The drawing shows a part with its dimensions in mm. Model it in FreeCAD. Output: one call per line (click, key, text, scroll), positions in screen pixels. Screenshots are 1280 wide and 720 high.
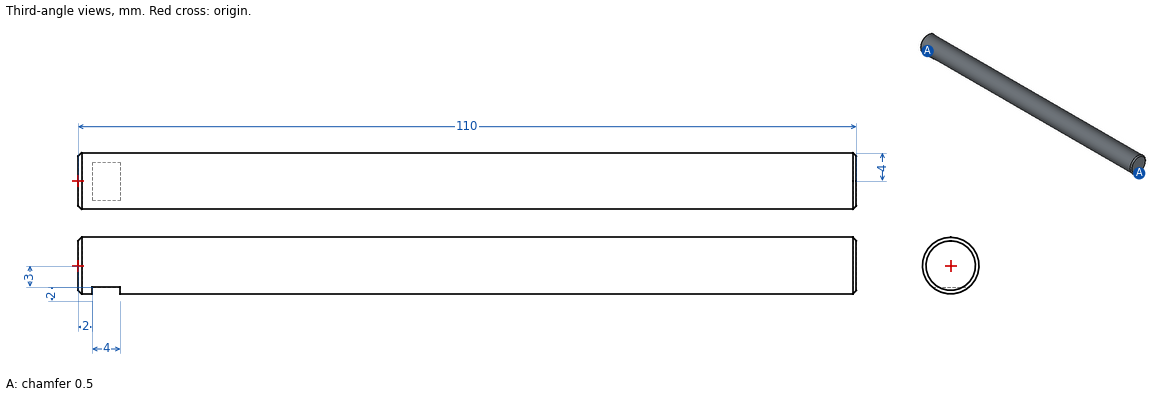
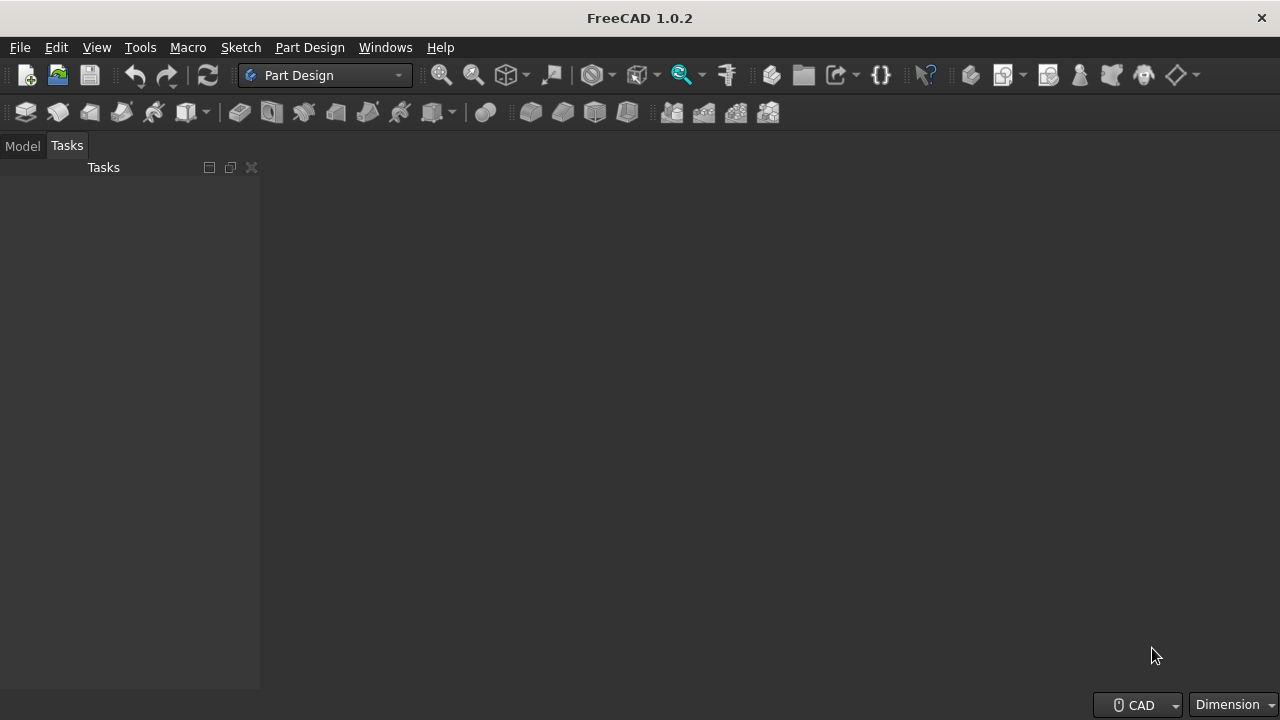
click(26, 76)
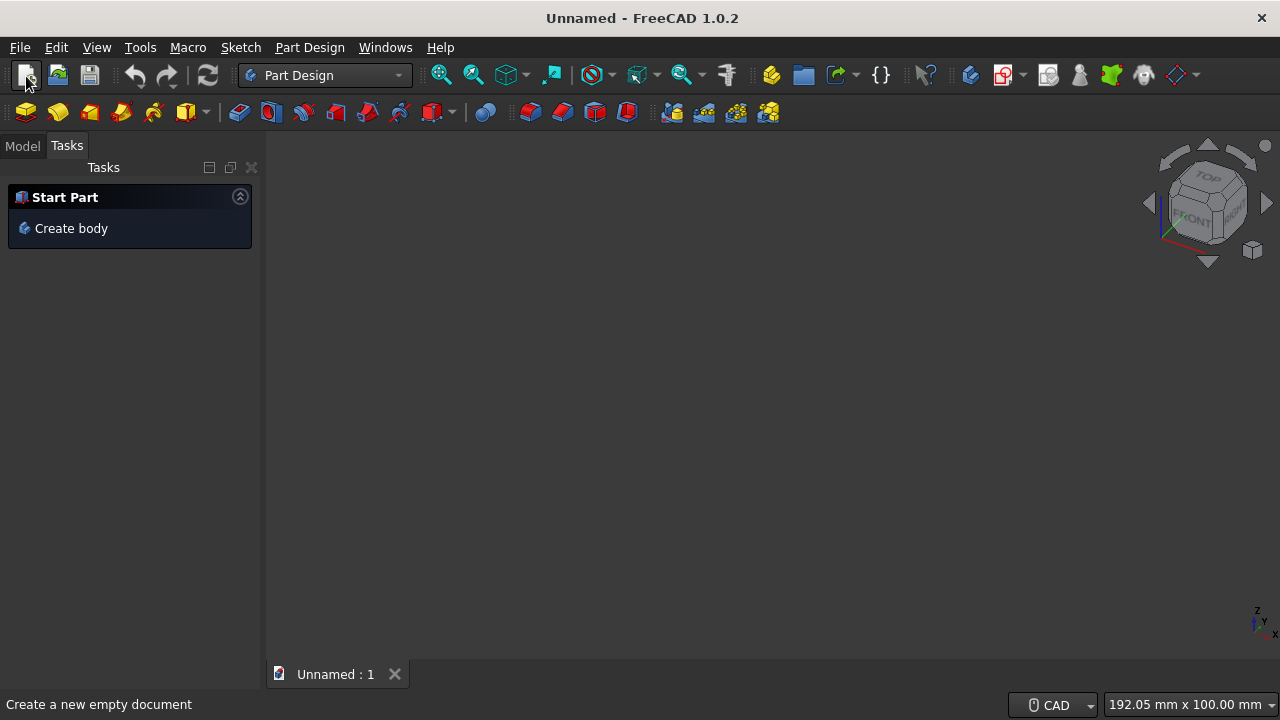
click(1004, 76)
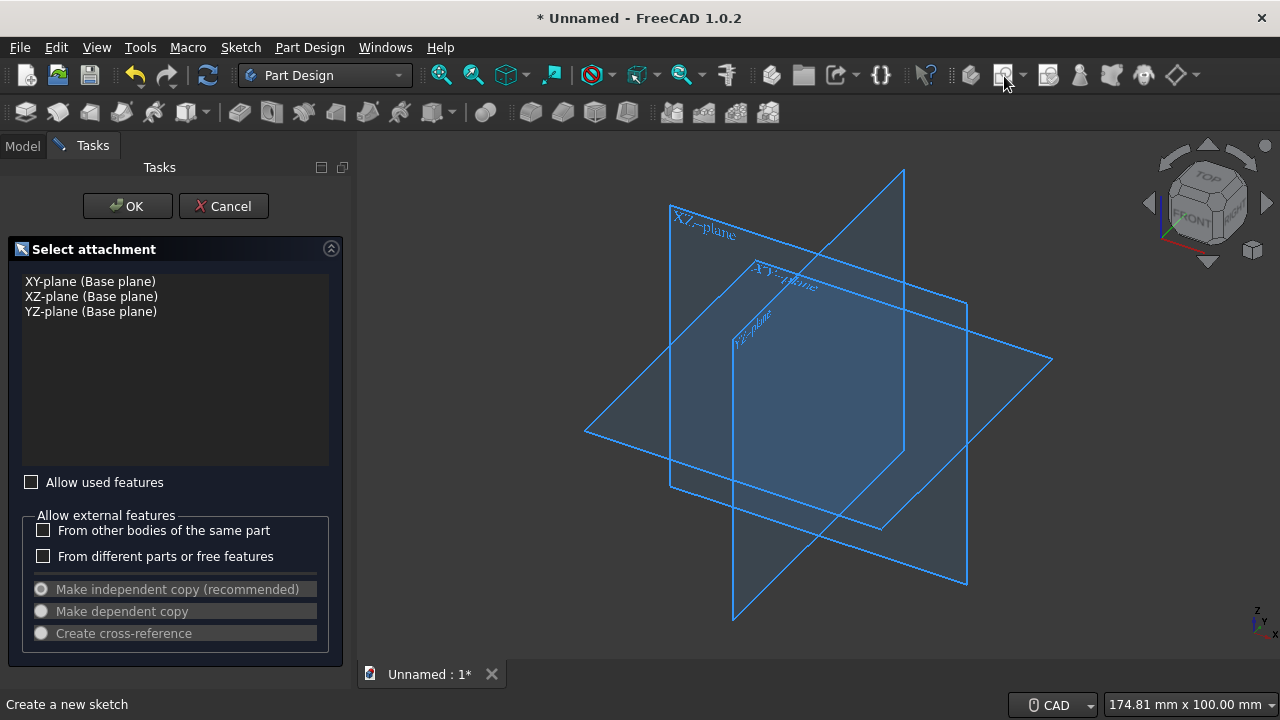
click(82, 282)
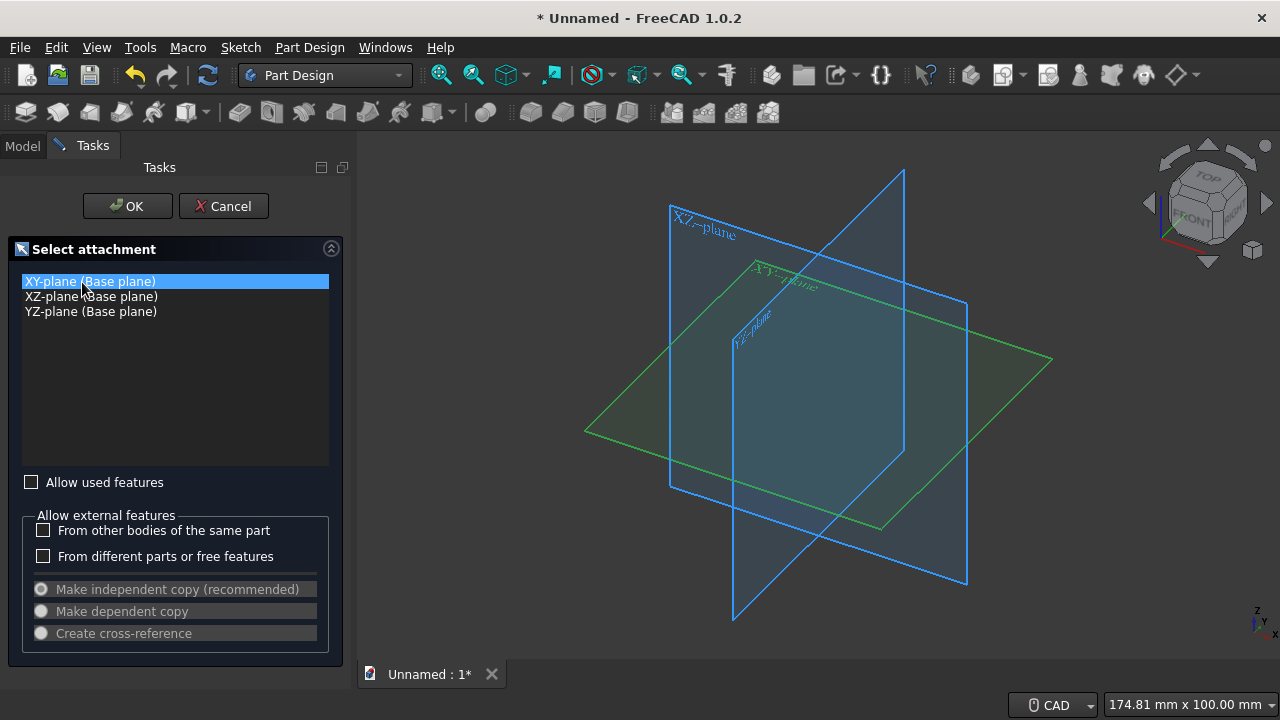
click(128, 206)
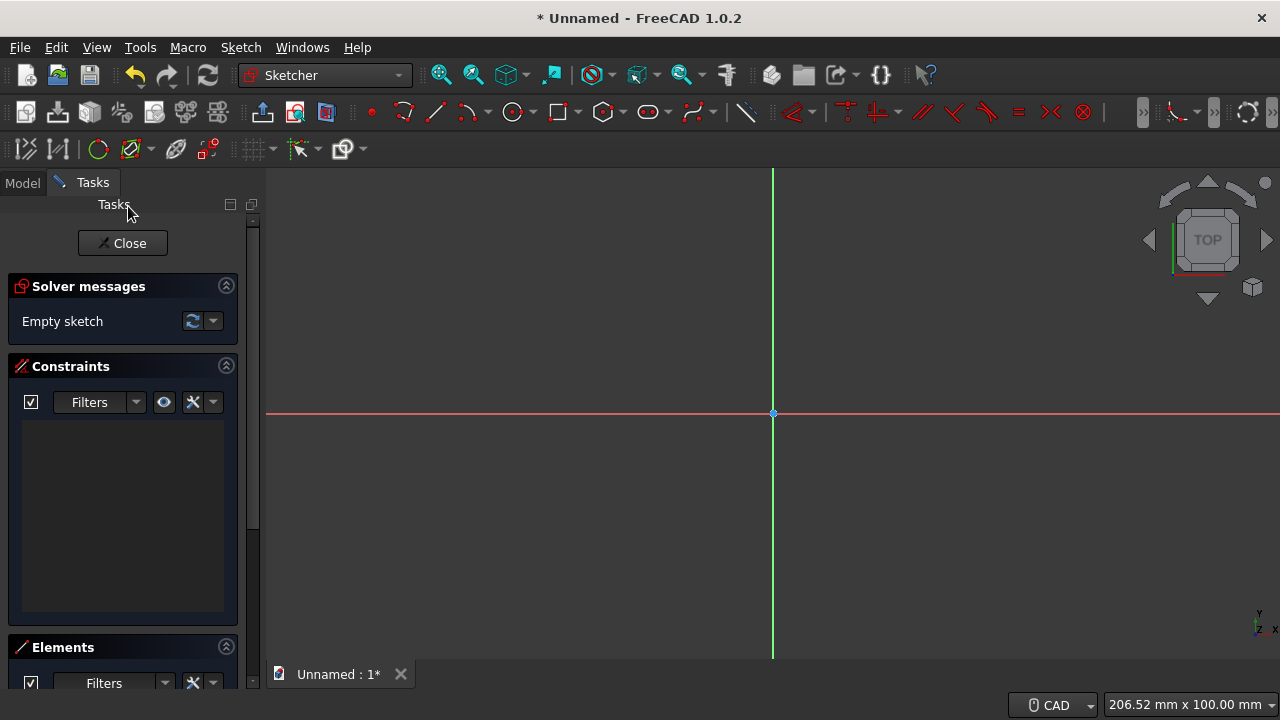
scroll(294, 433, down, 2)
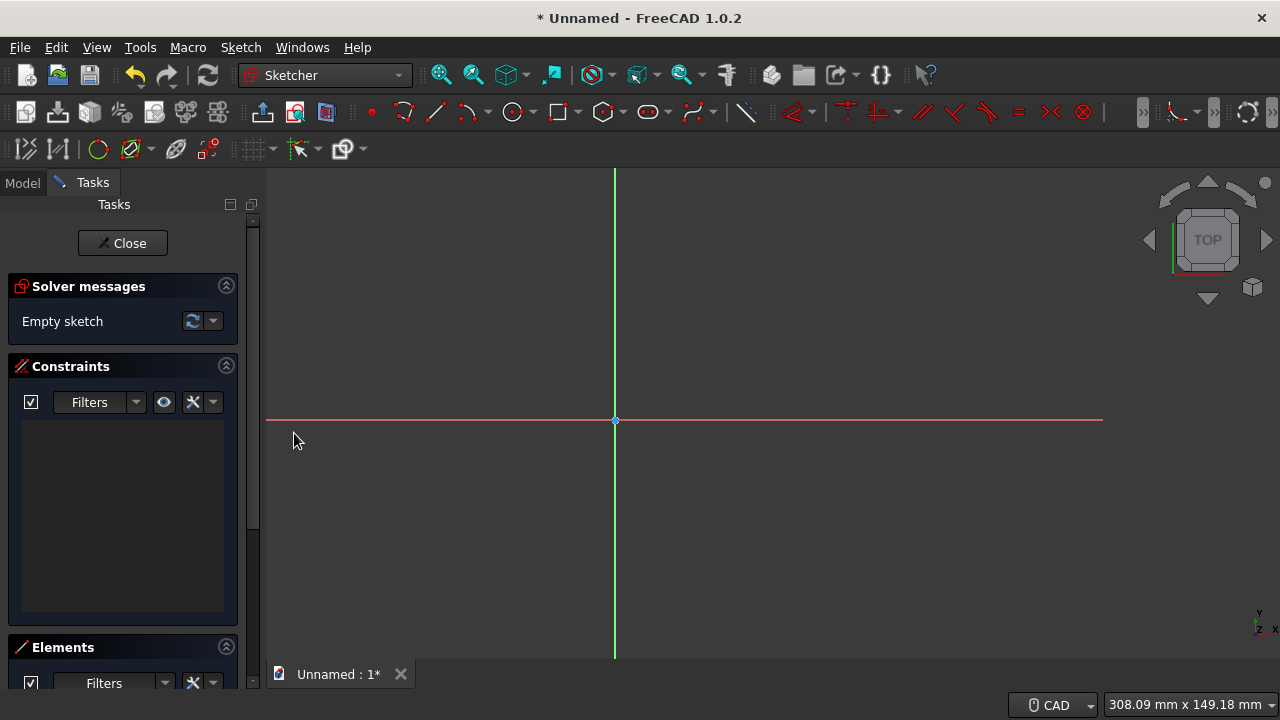
scroll(982, 414, up, 2)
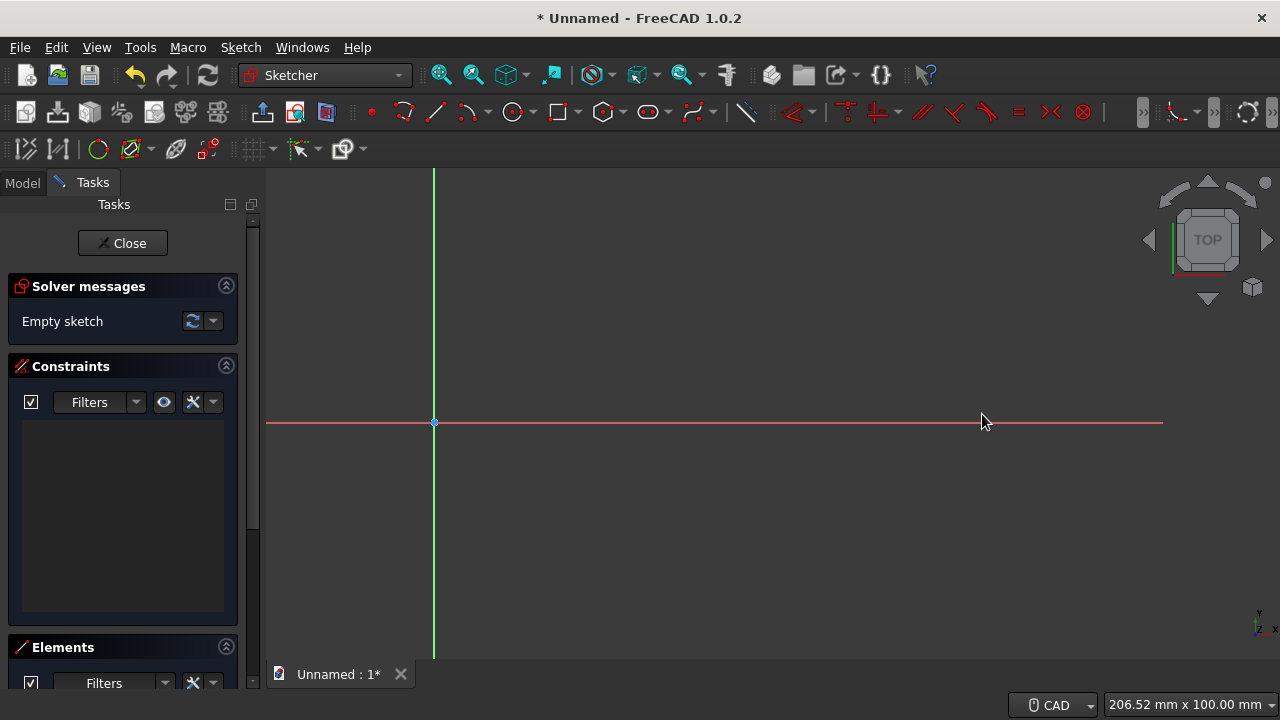
click(558, 112)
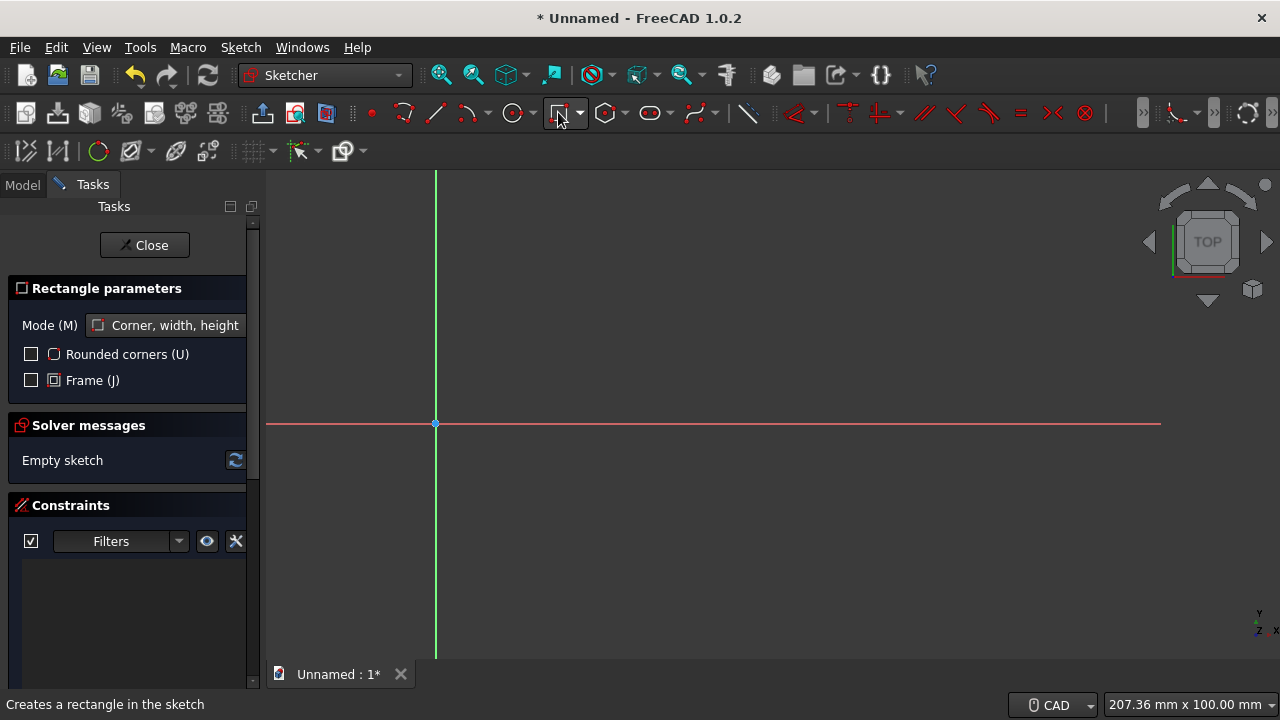
click(436, 424)
click(974, 404)
key(Escape)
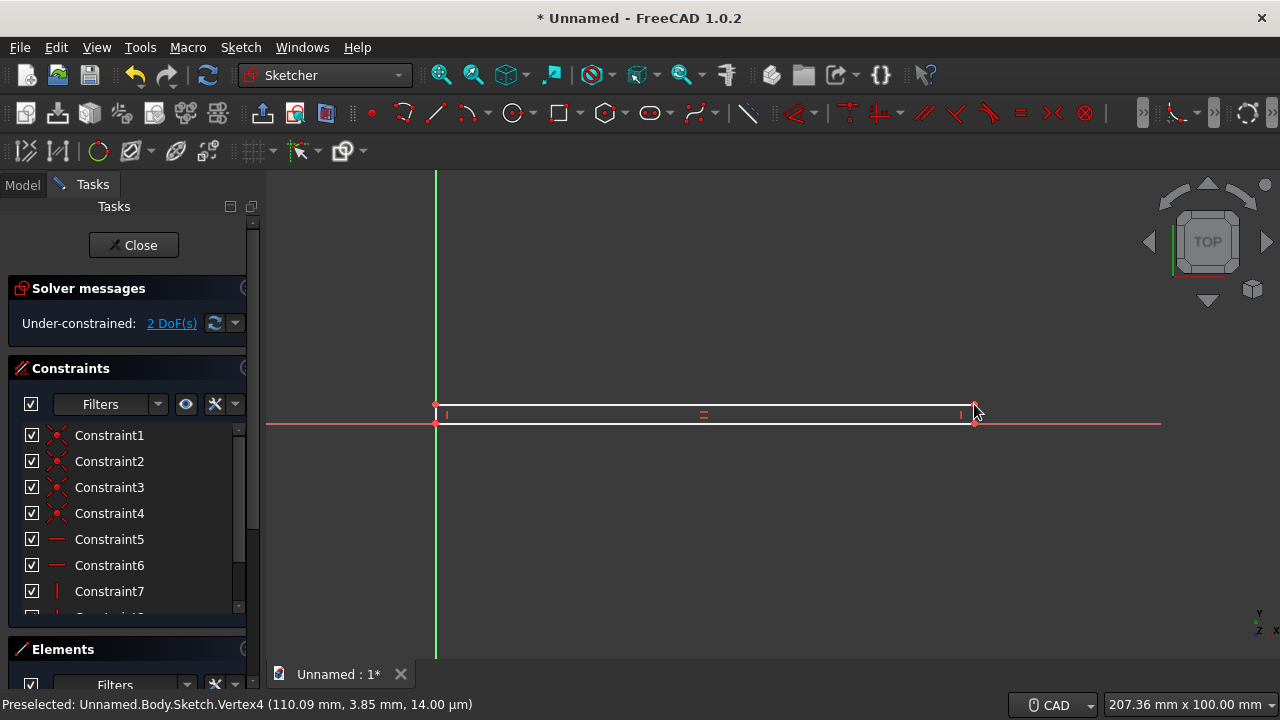
key(d)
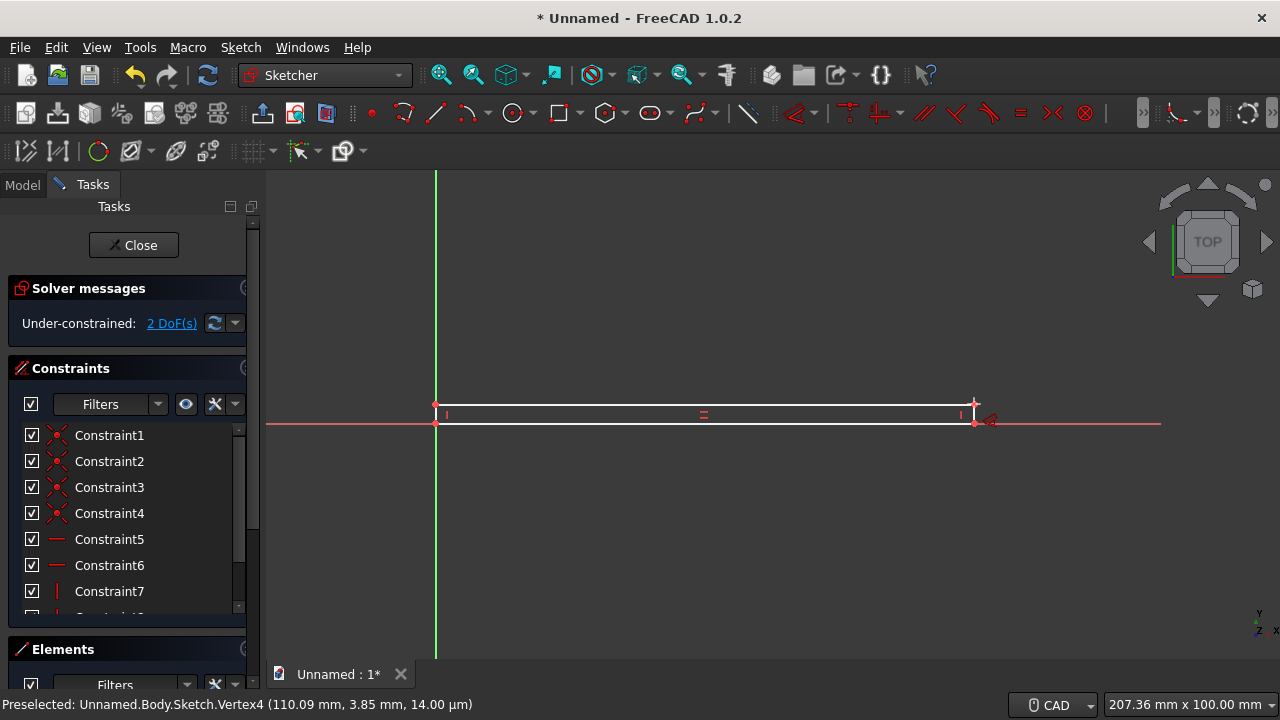
scroll(974, 414, up, 4)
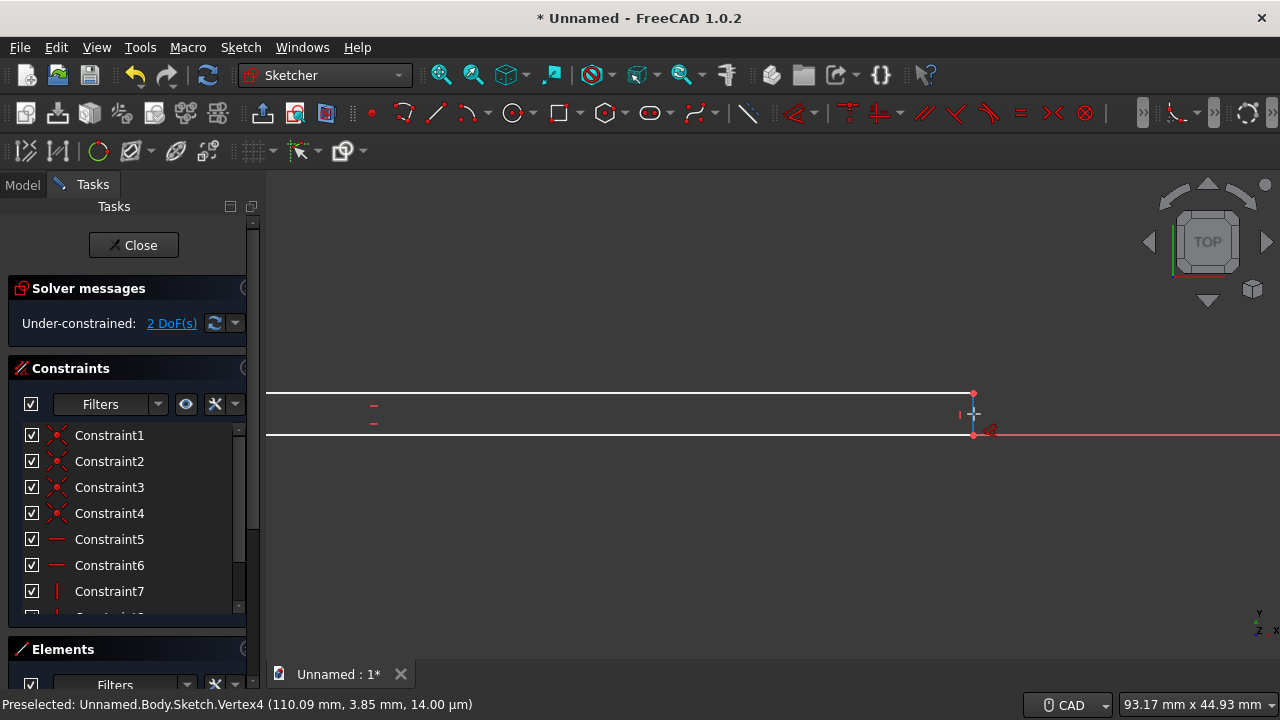
click(973, 414)
click(1007, 414)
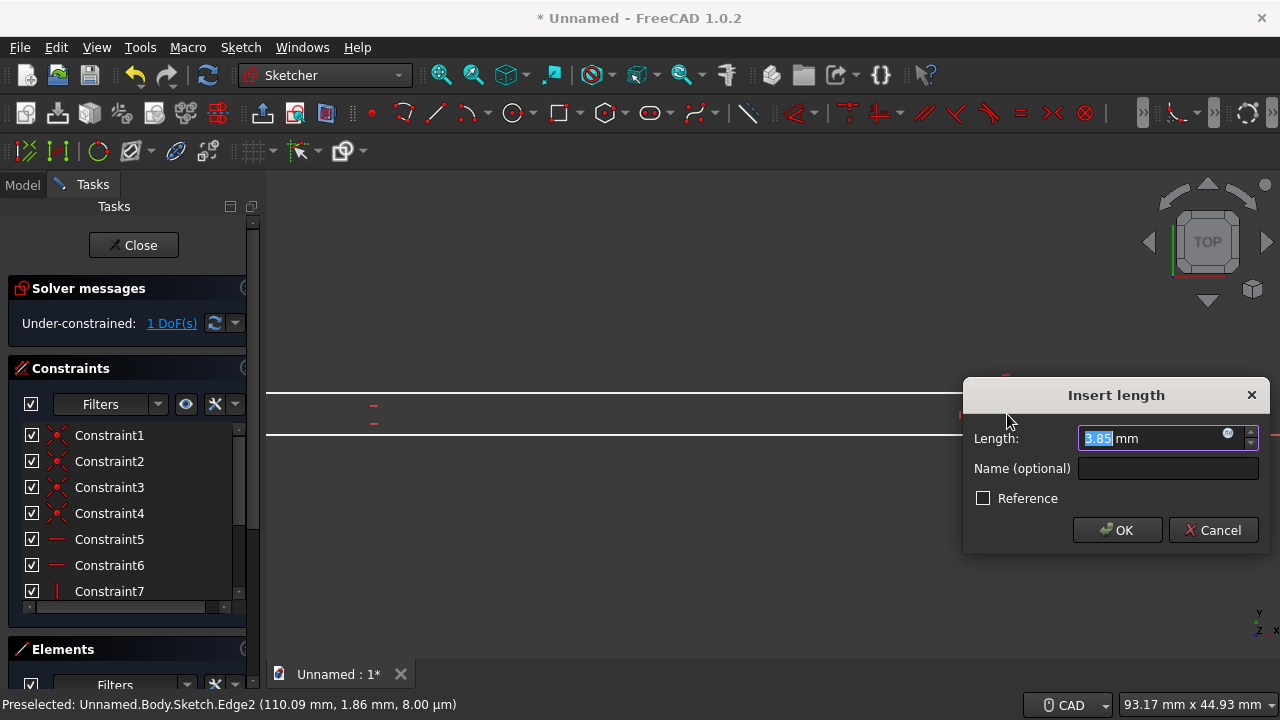
text(4)
key(Return)